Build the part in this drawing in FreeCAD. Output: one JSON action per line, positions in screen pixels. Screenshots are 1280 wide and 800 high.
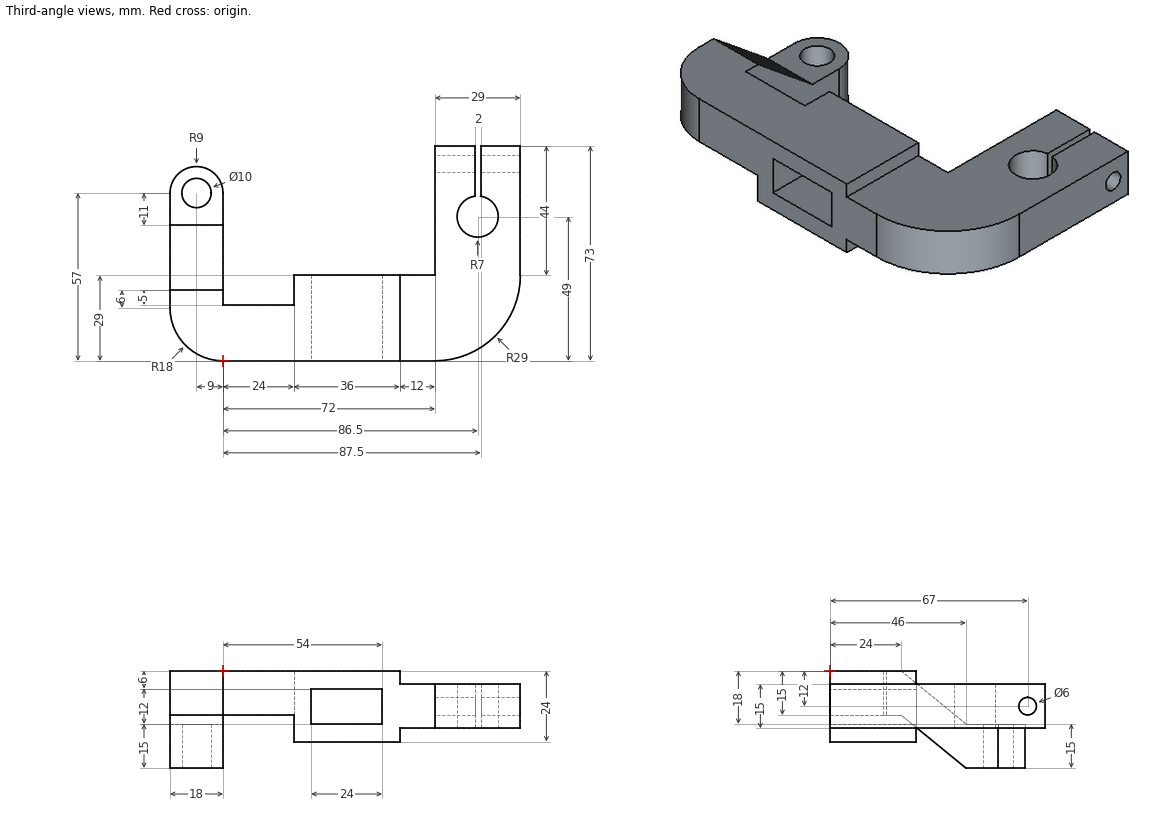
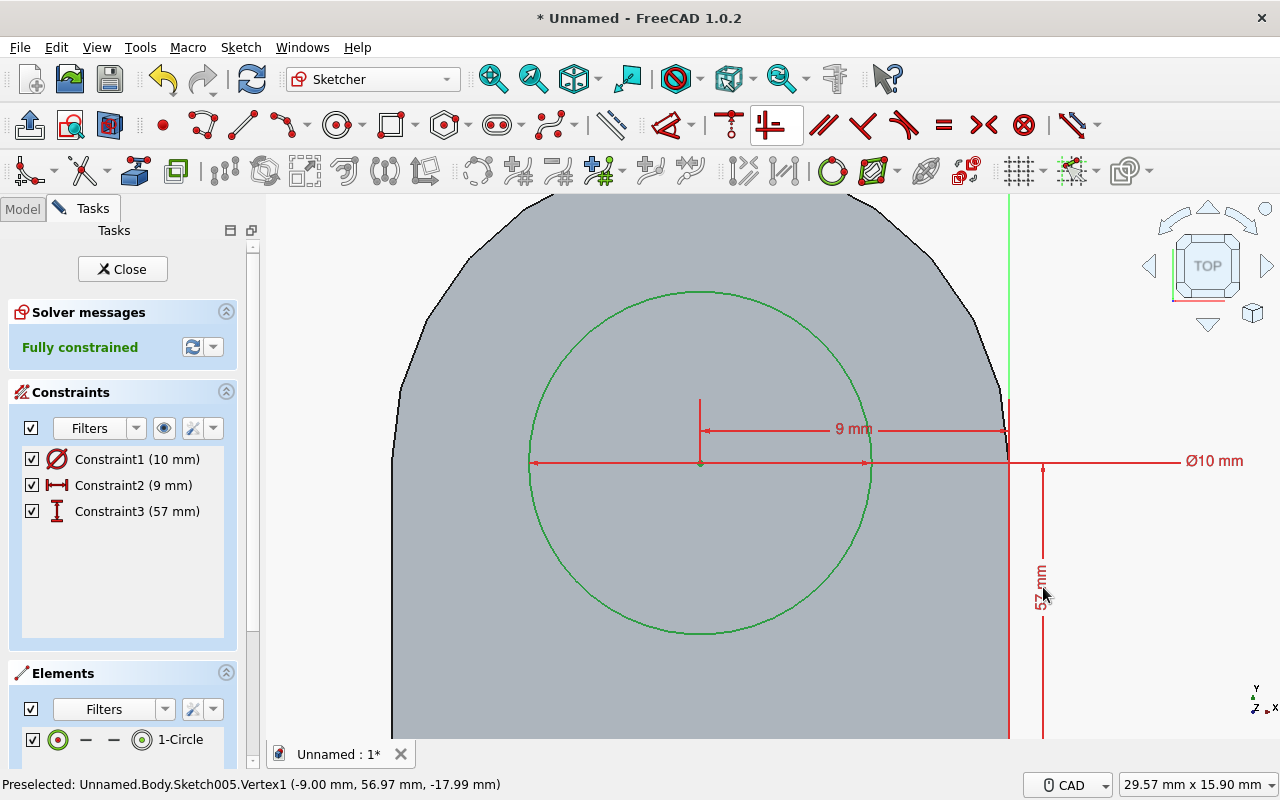
{"action": "left_click", "coordinate": [123, 269]}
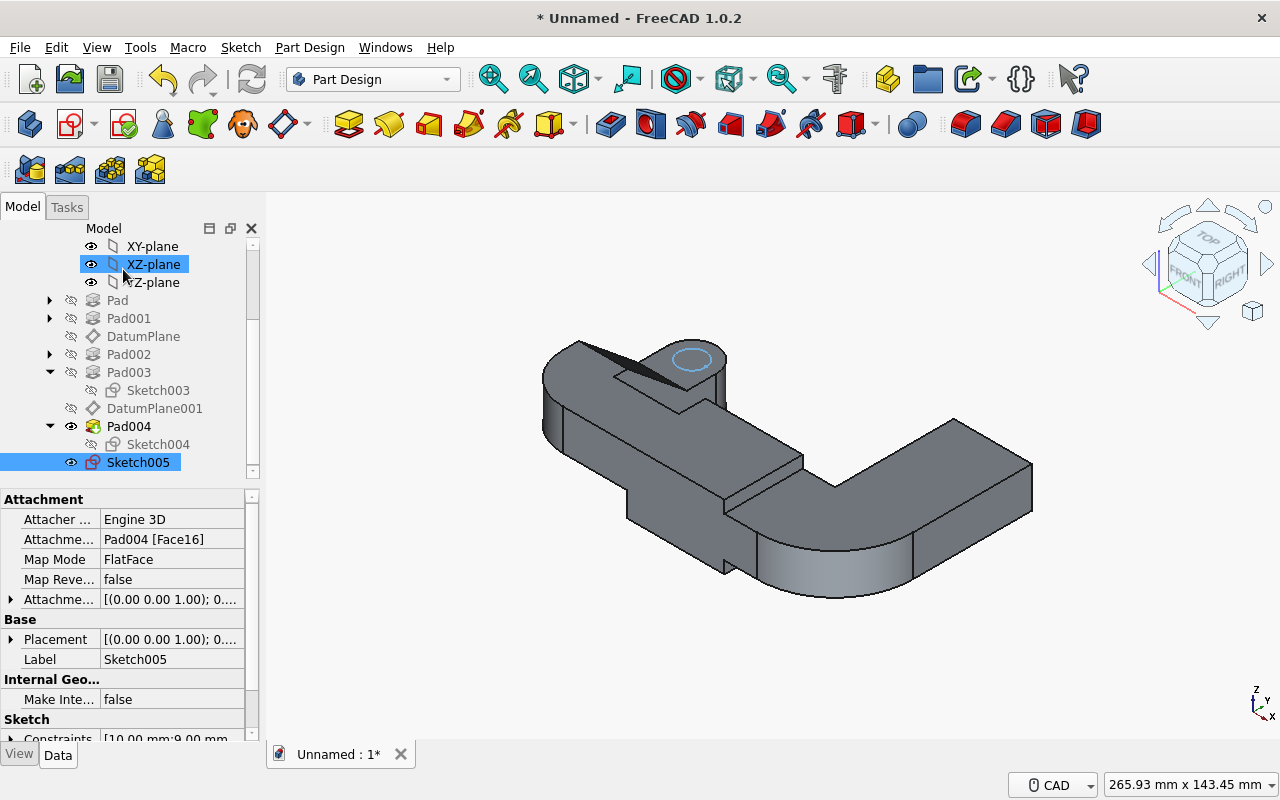
{"action": "left_click", "coordinate": [612, 124]}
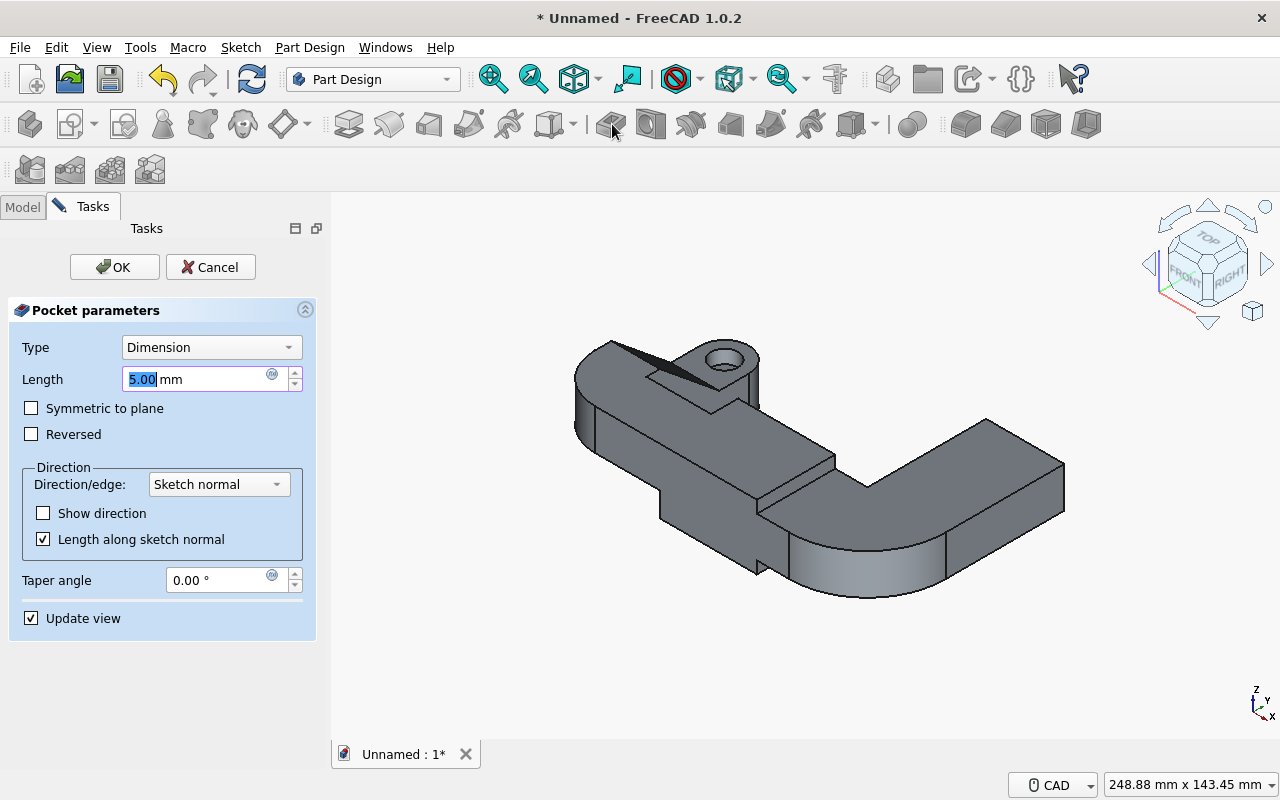
{"action": "type", "text": "15"}
{"action": "key", "text": "Tab"}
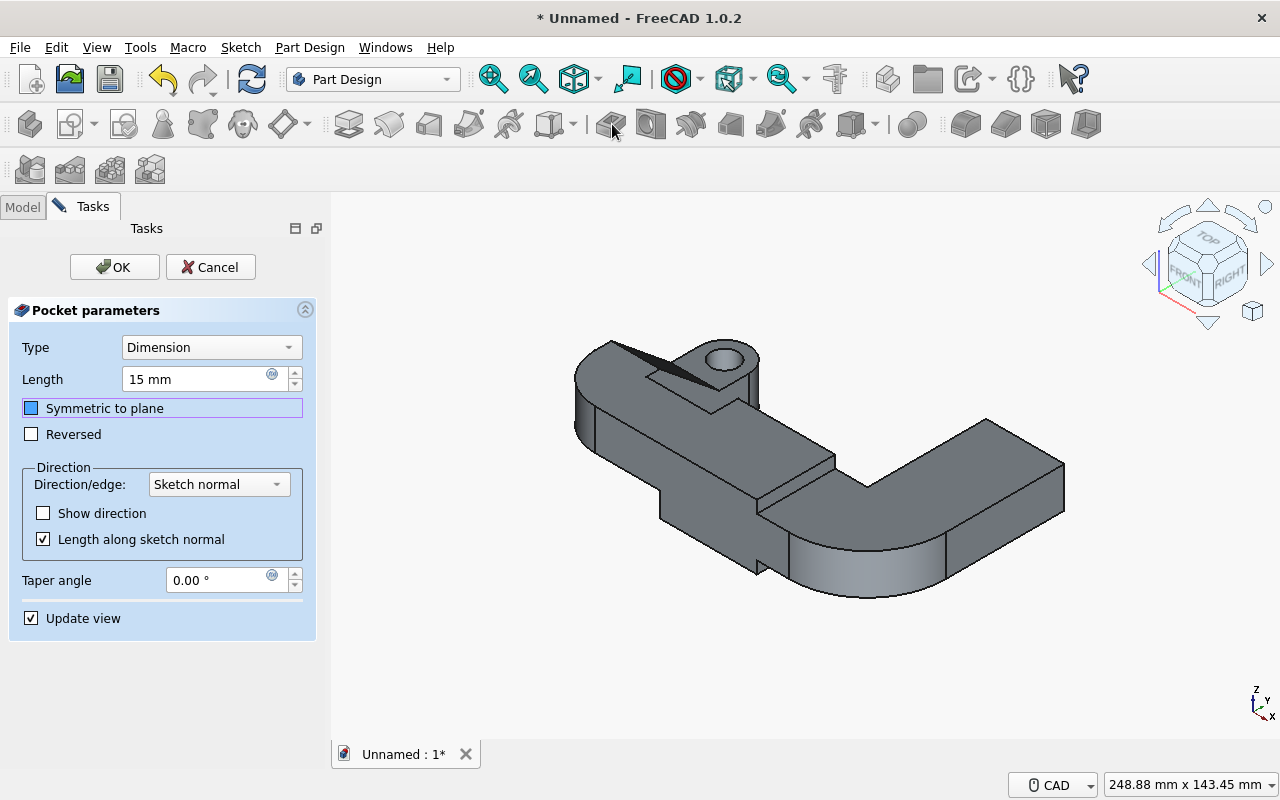
{"action": "left_click", "coordinate": [115, 267]}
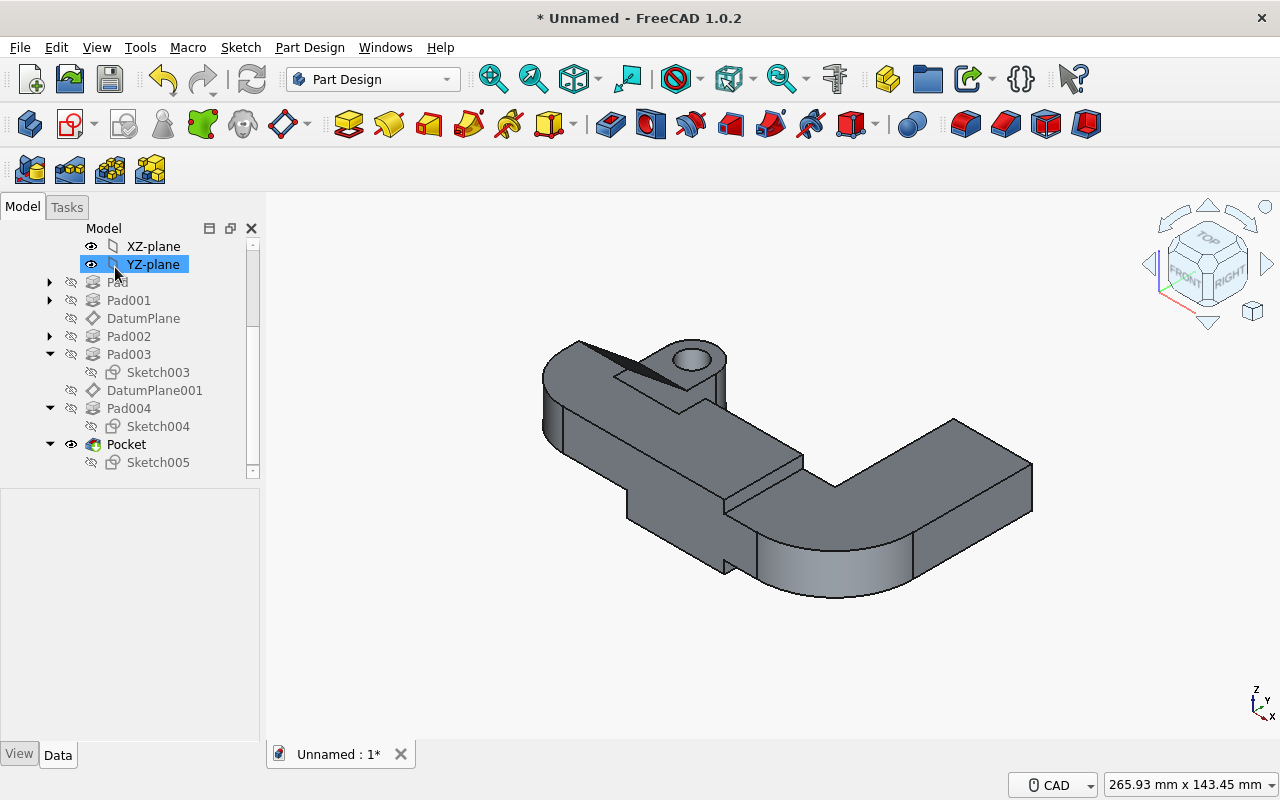
{"action": "key", "text": "4"}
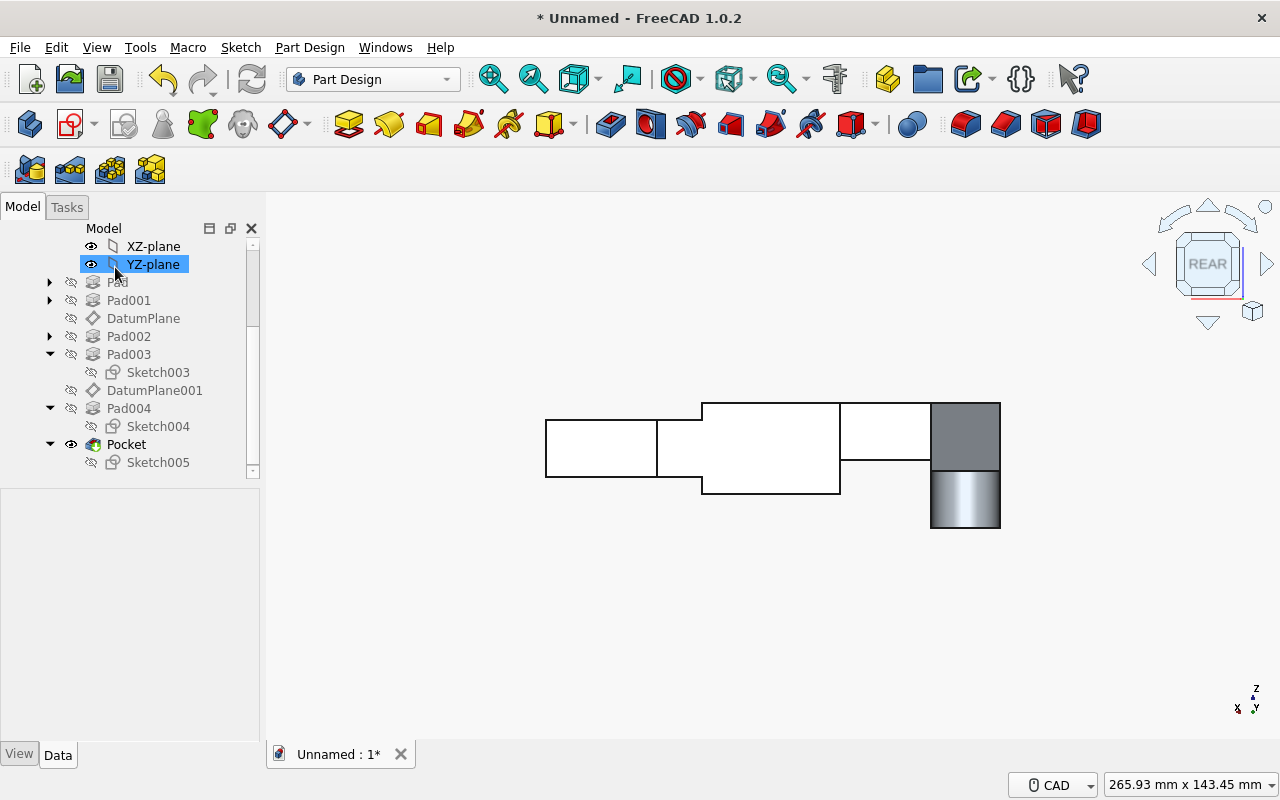
{"action": "left_click", "coordinate": [494, 80]}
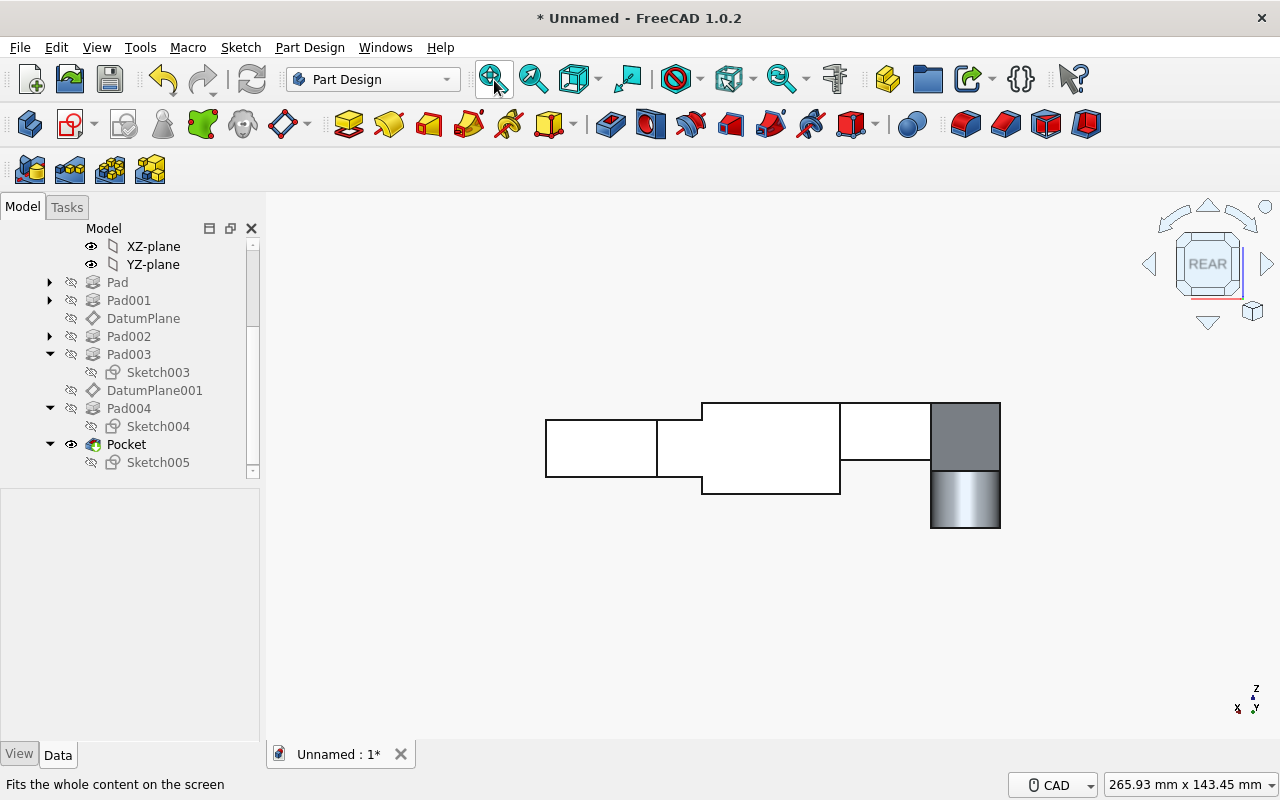
{"action": "left_click", "coordinate": [748, 447]}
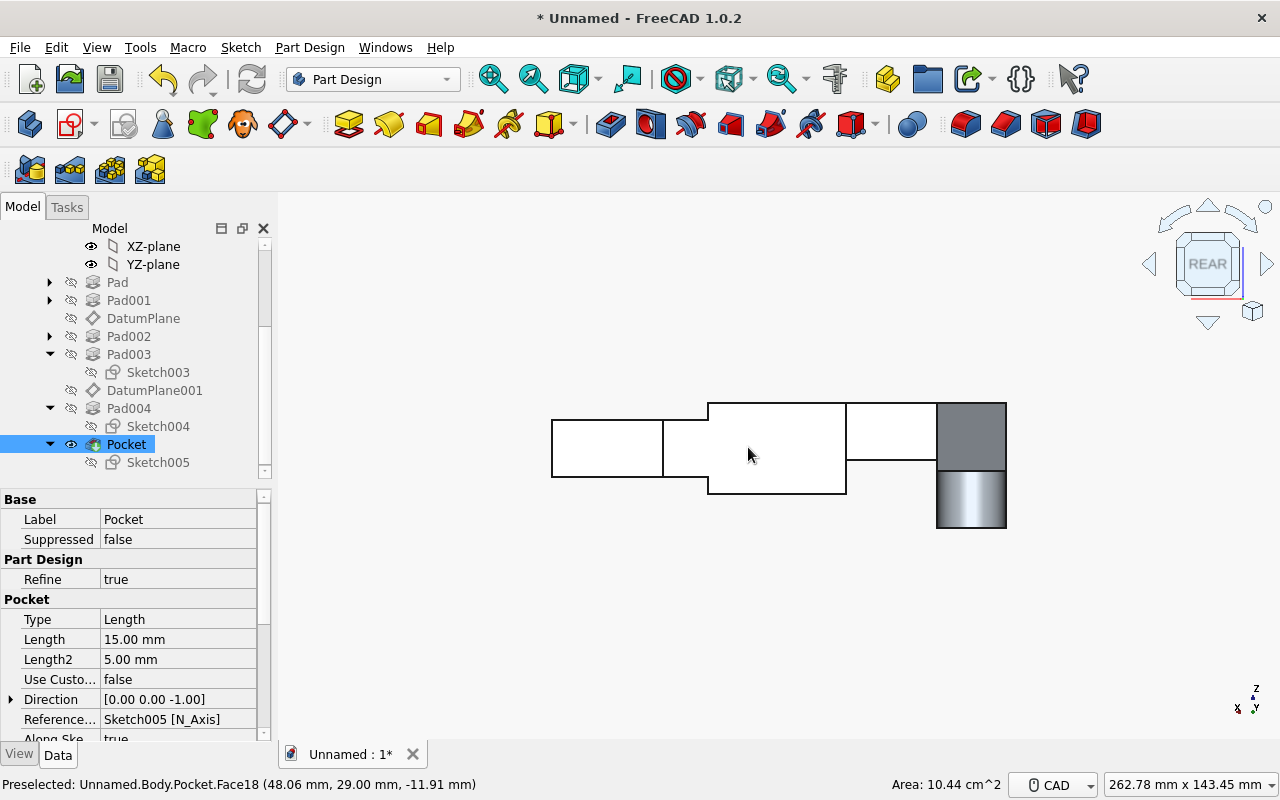
{"action": "left_click", "coordinate": [70, 124]}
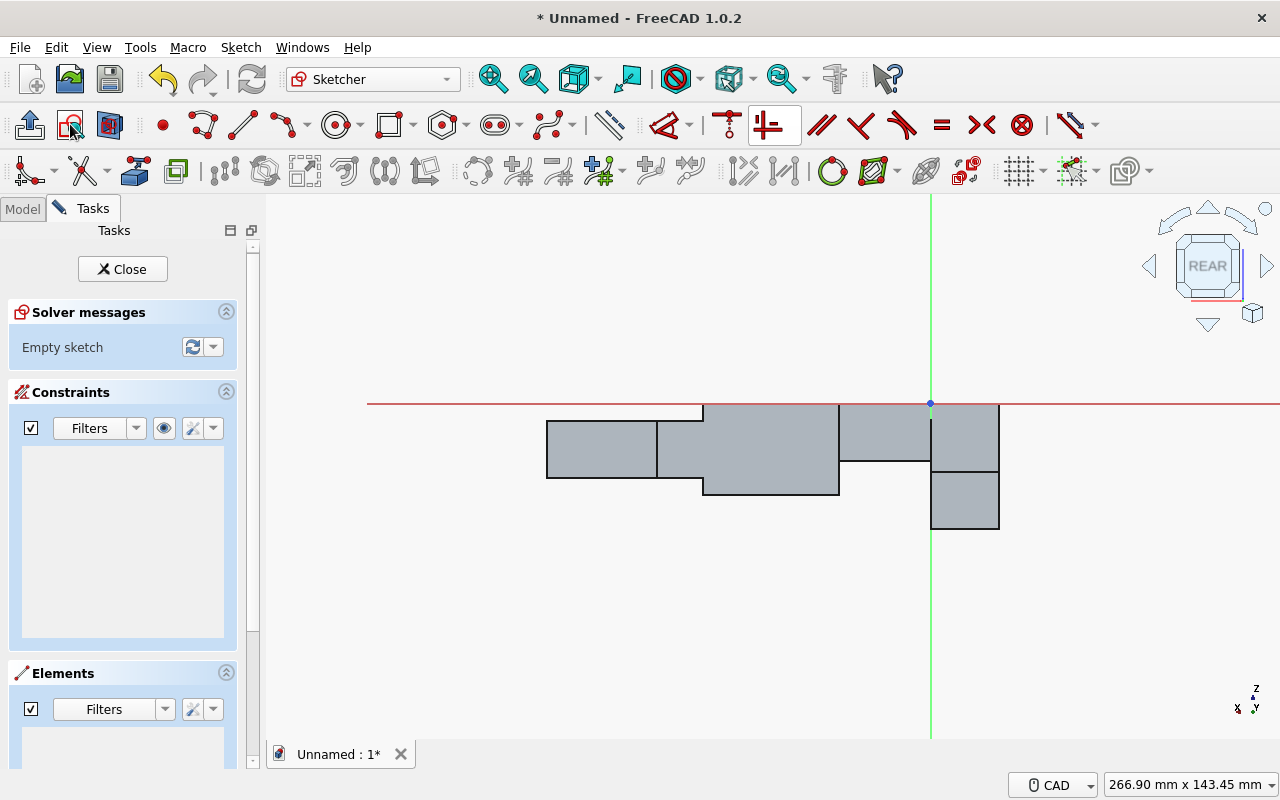
{"action": "left_click", "coordinate": [110, 126]}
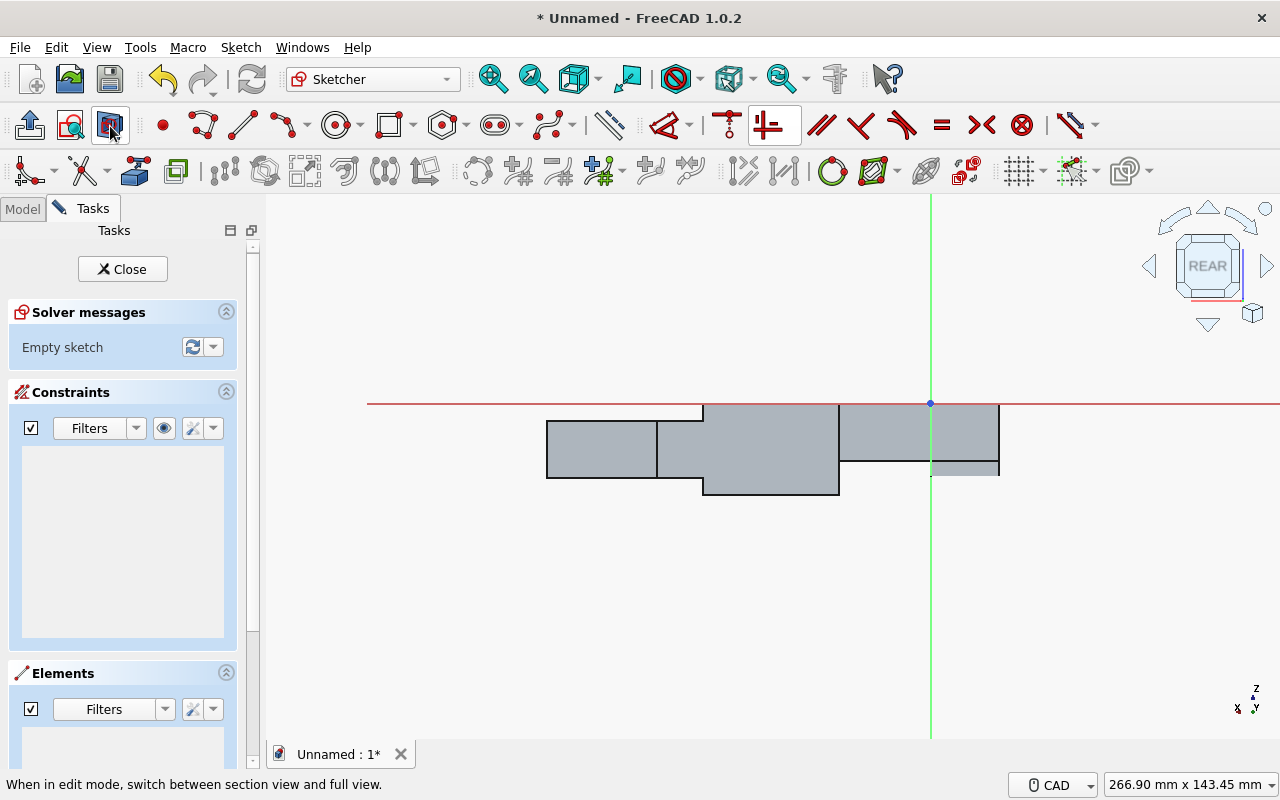
{"action": "scroll", "coordinate": [900, 421], "scroll_direction": "up", "scroll_amount": 5}